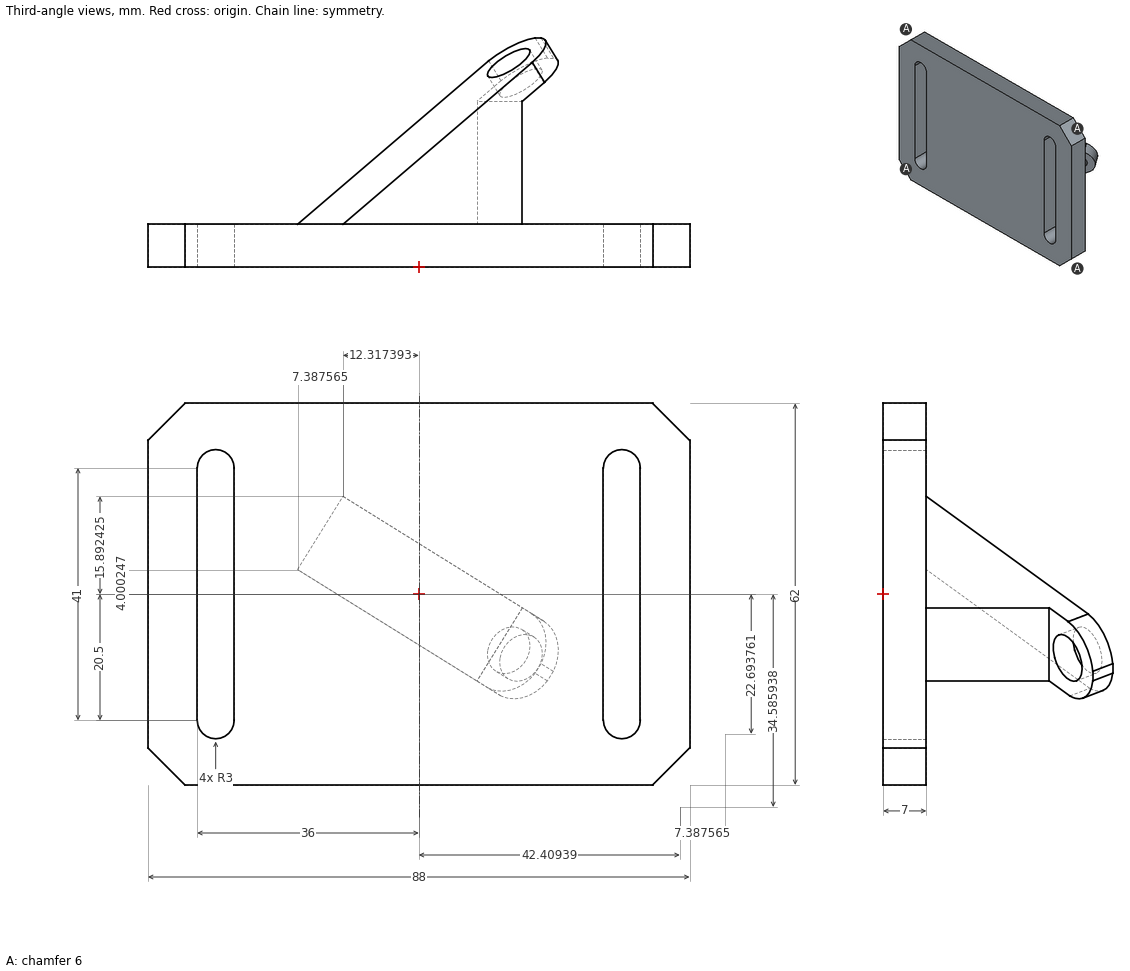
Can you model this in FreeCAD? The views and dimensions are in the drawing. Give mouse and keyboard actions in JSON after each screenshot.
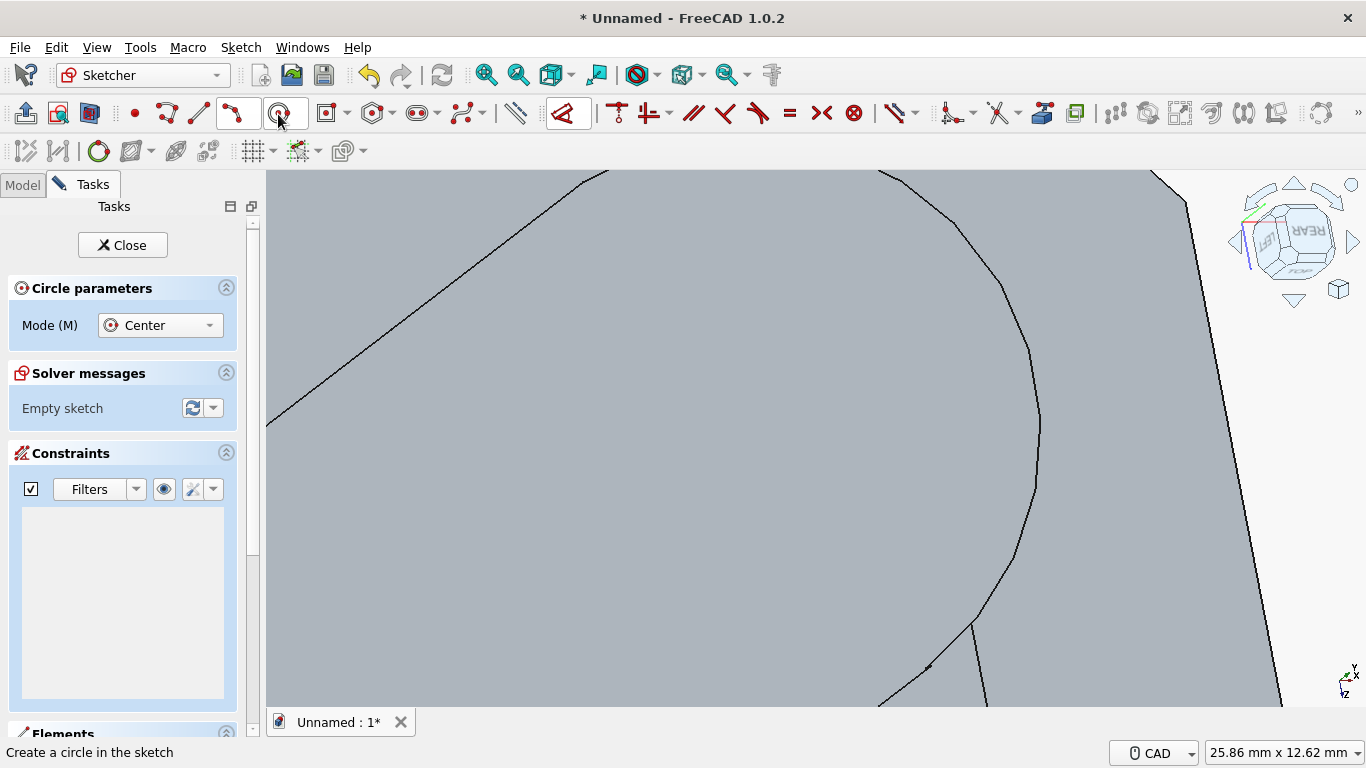
{"action": "left_click", "coordinate": [743, 434]}
{"action": "mouse_move", "coordinate": [863, 313]}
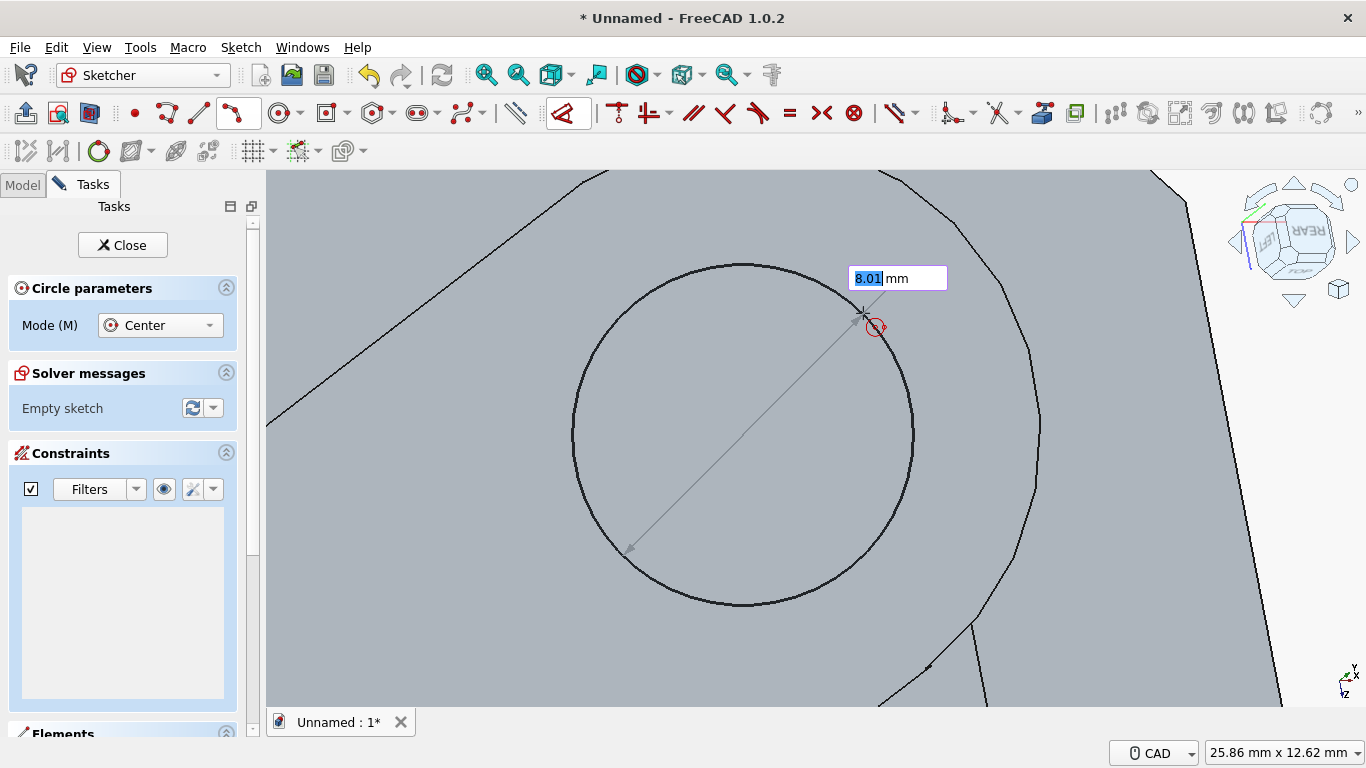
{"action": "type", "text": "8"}
{"action": "key", "text": "Return"}
{"action": "key", "text": "Escape"}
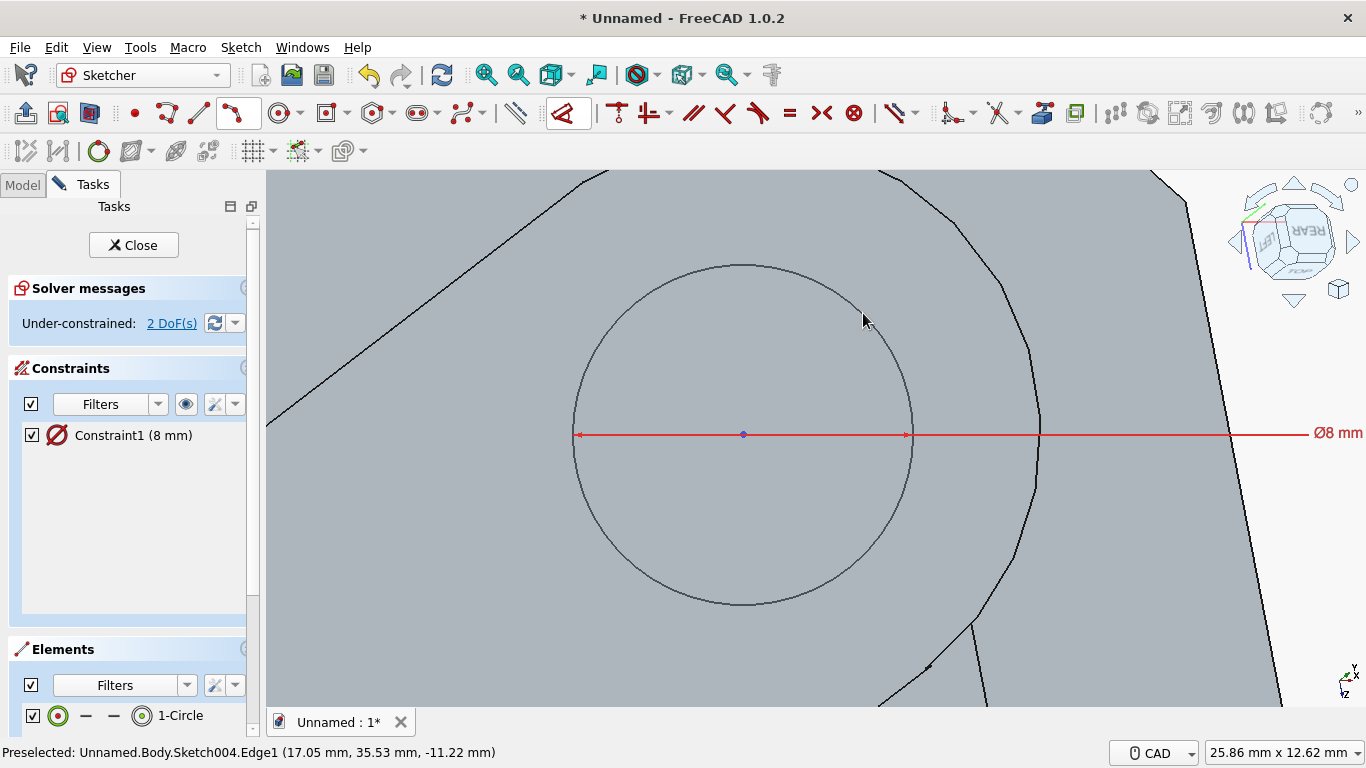
{"action": "left_click", "coordinate": [743, 435]}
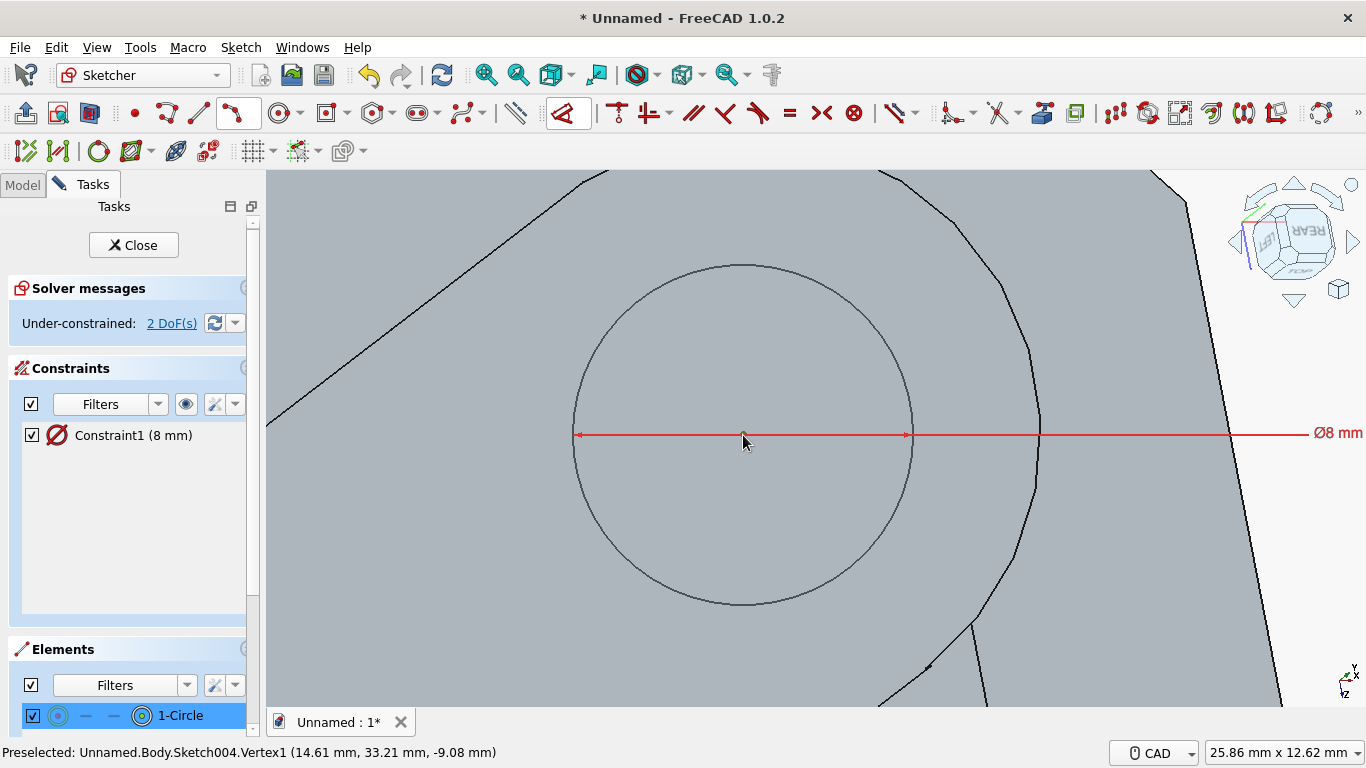
{"action": "left_click", "coordinate": [586, 114]}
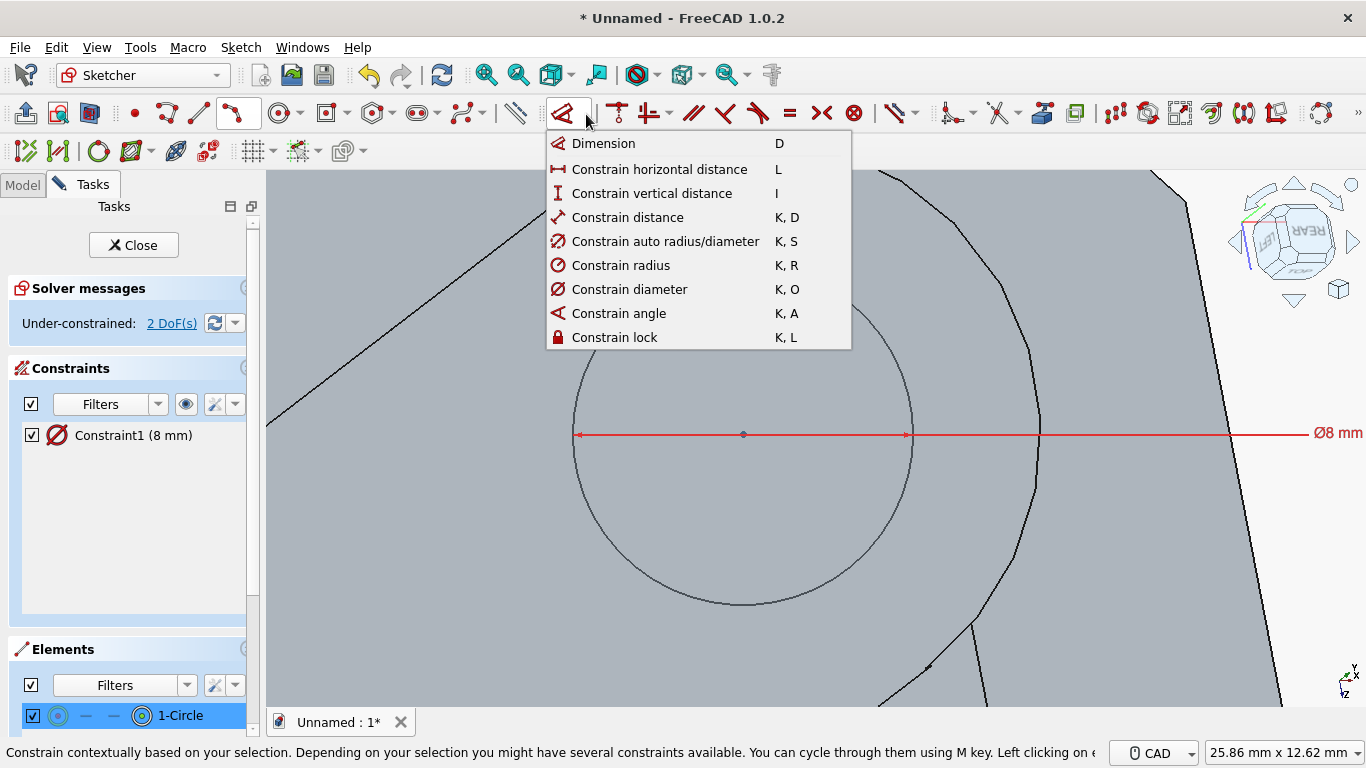
{"action": "left_click", "coordinate": [699, 169]}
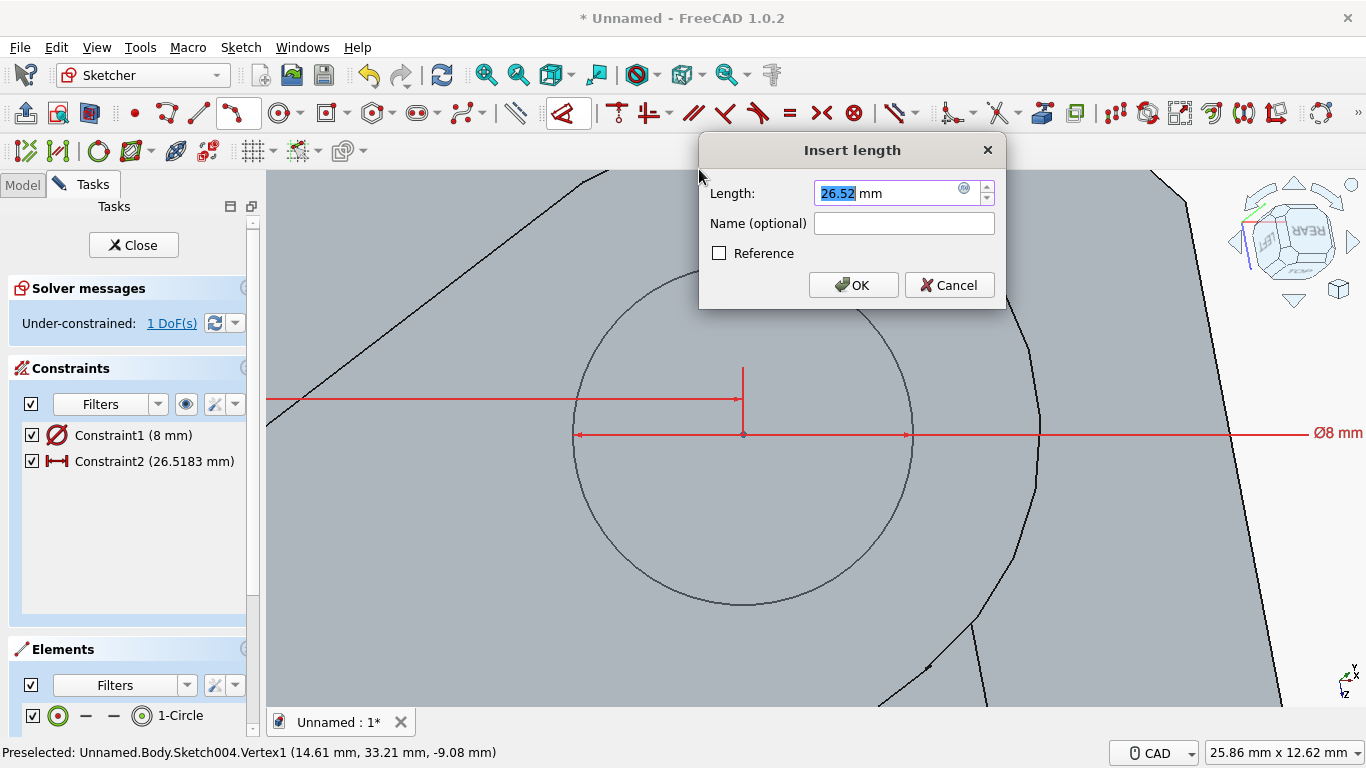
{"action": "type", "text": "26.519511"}
{"action": "key", "text": "Return"}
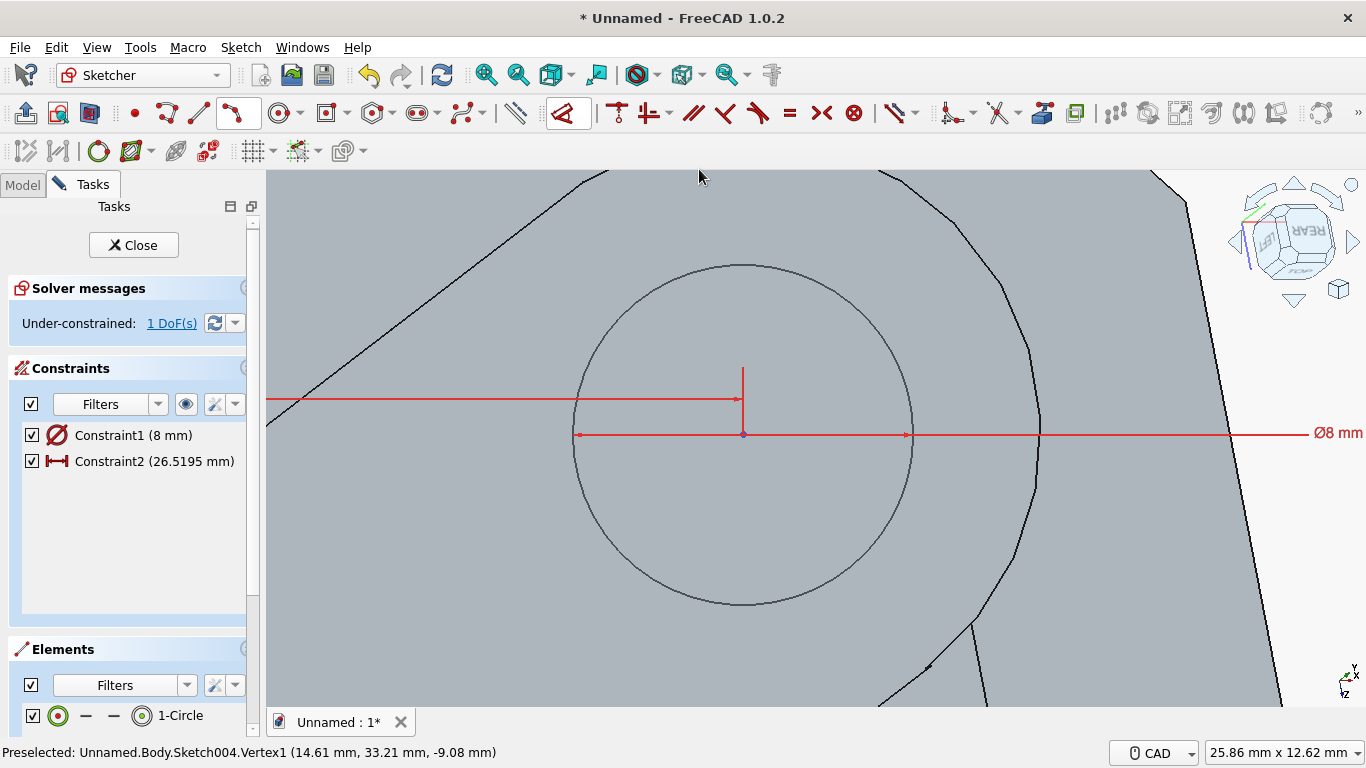
{"action": "left_click", "coordinate": [743, 435]}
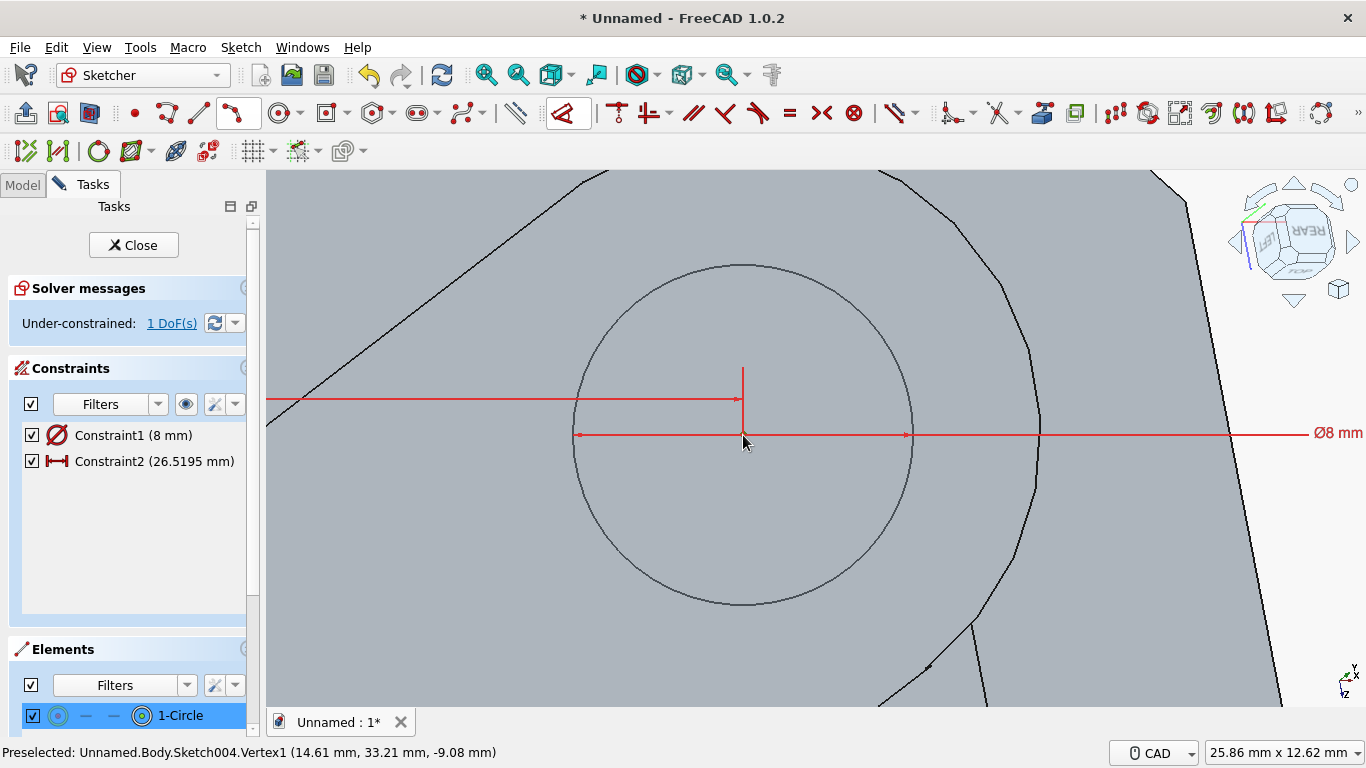
{"action": "left_click", "coordinate": [586, 114]}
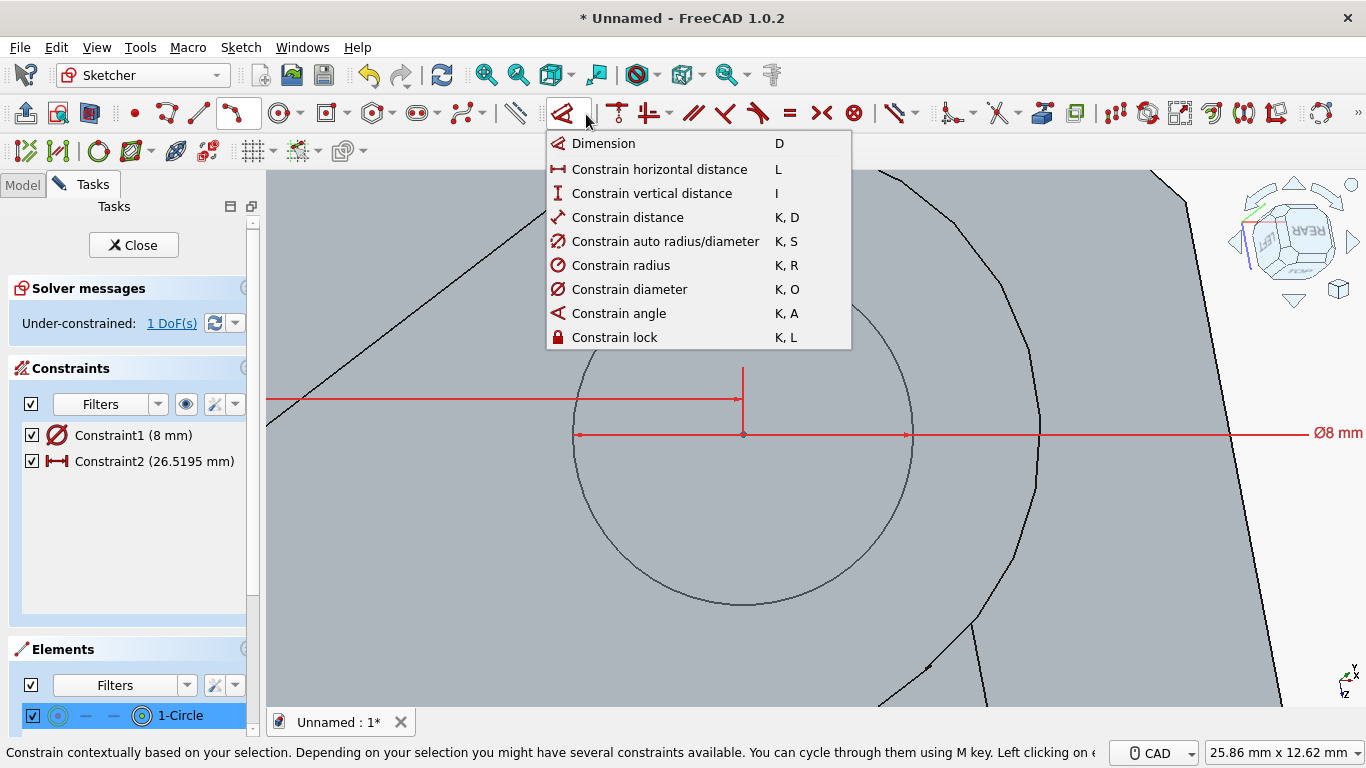
{"action": "left_click", "coordinate": [699, 193]}